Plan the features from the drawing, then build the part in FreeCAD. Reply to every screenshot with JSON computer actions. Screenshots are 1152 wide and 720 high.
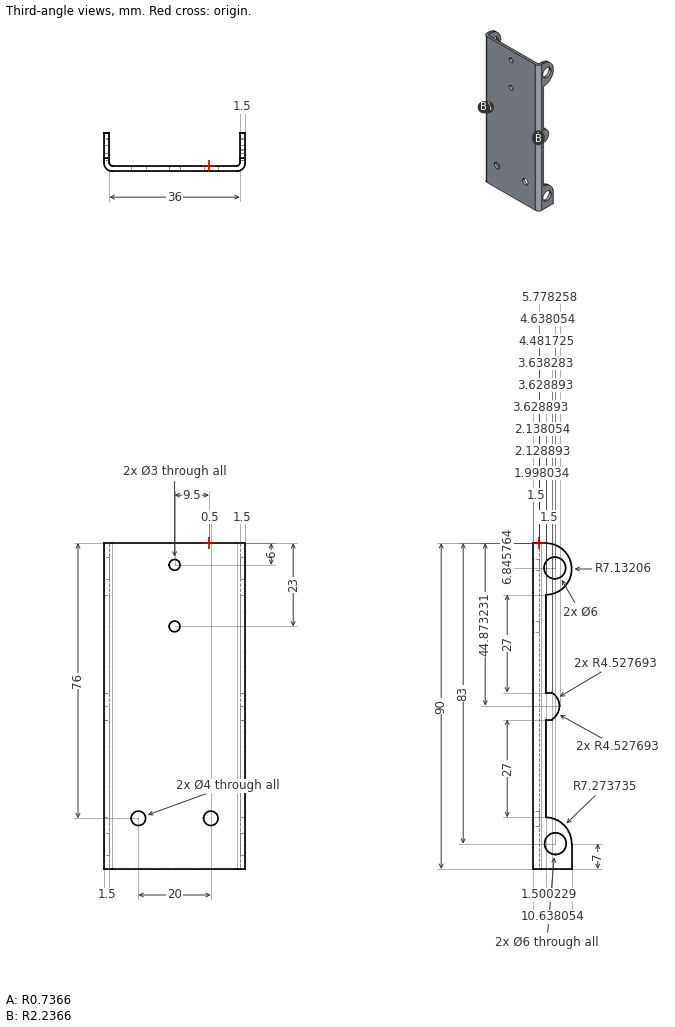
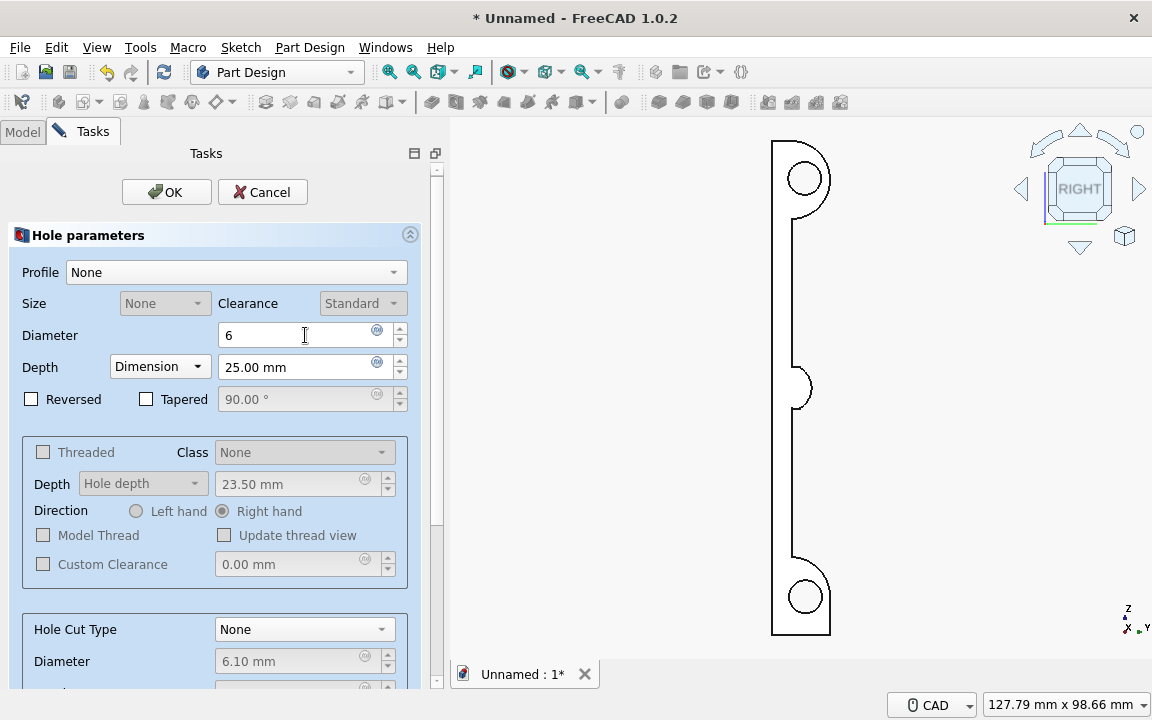
{"action": "left_click", "coordinate": [161, 366]}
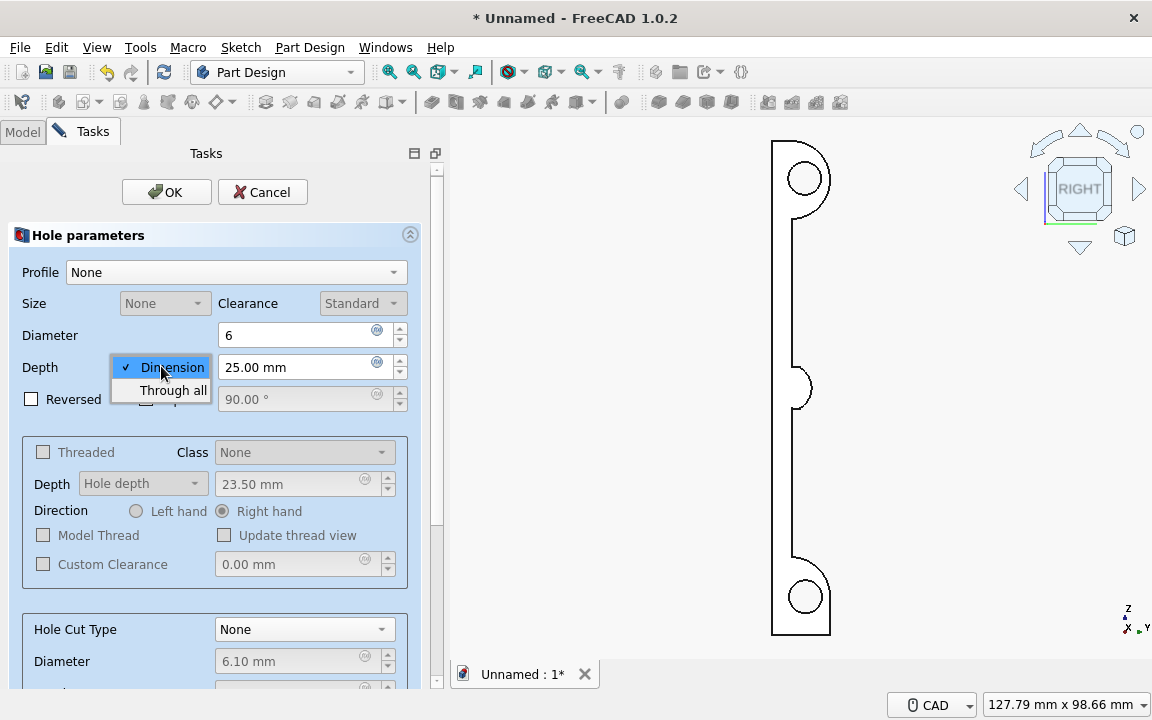
{"action": "left_click", "coordinate": [160, 390]}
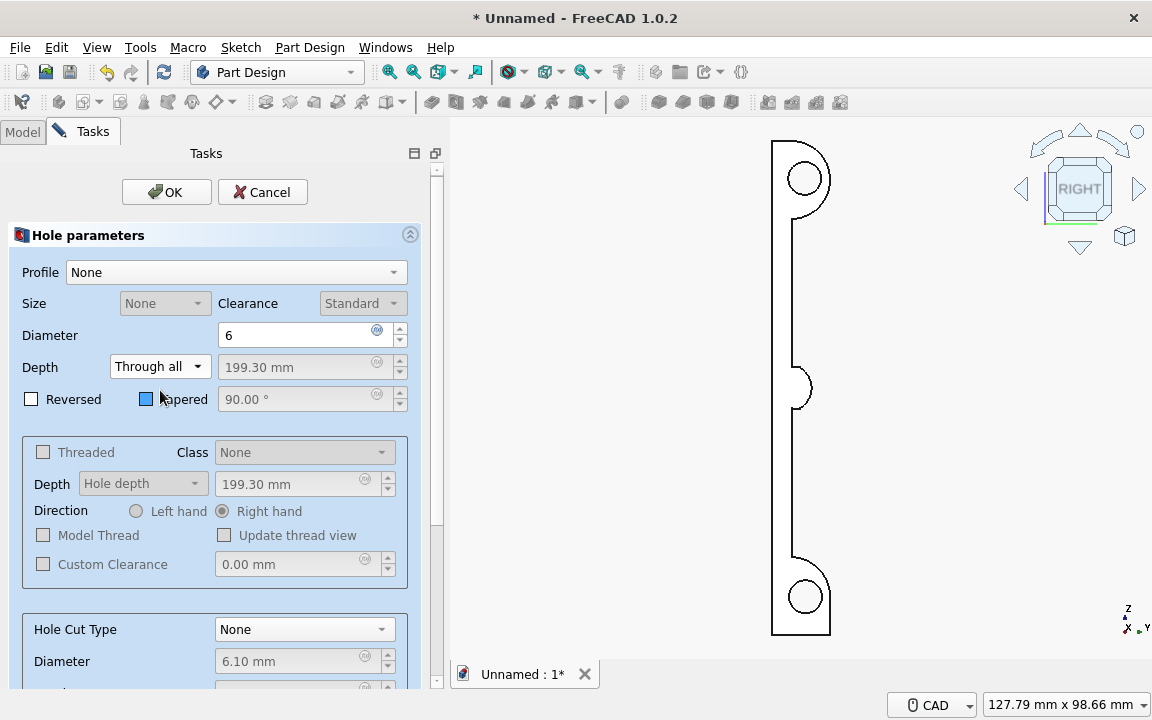
{"action": "left_click", "coordinate": [167, 192]}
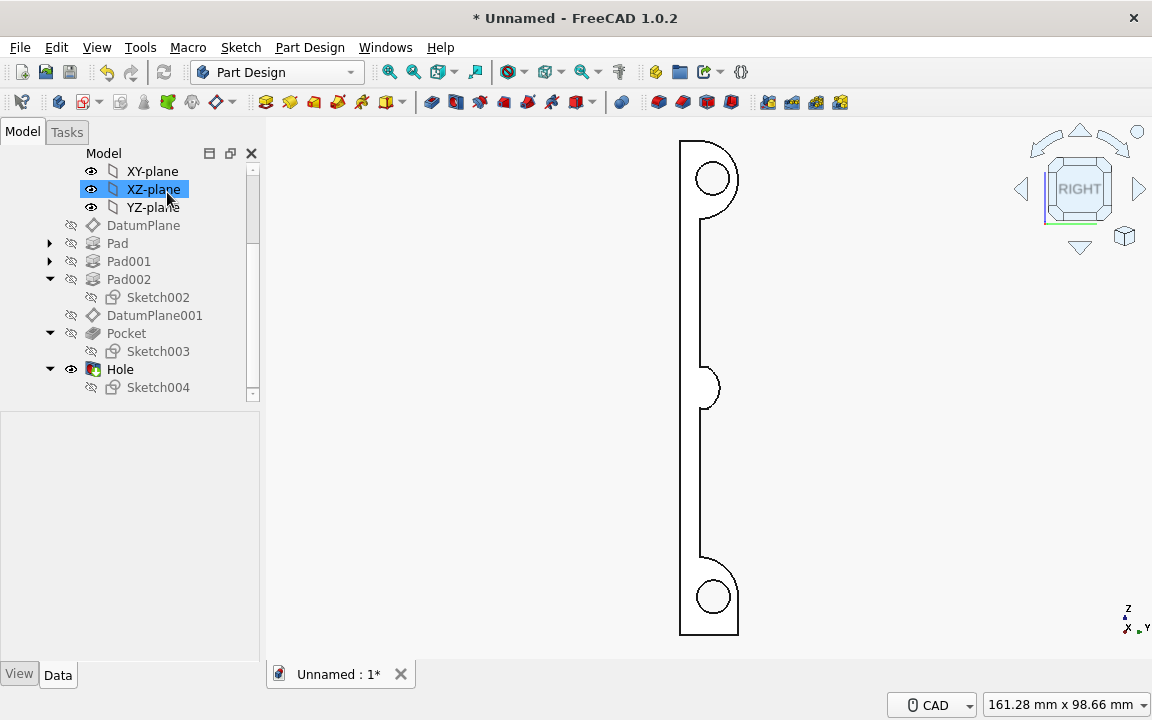
{"action": "left_click", "coordinate": [84, 102]}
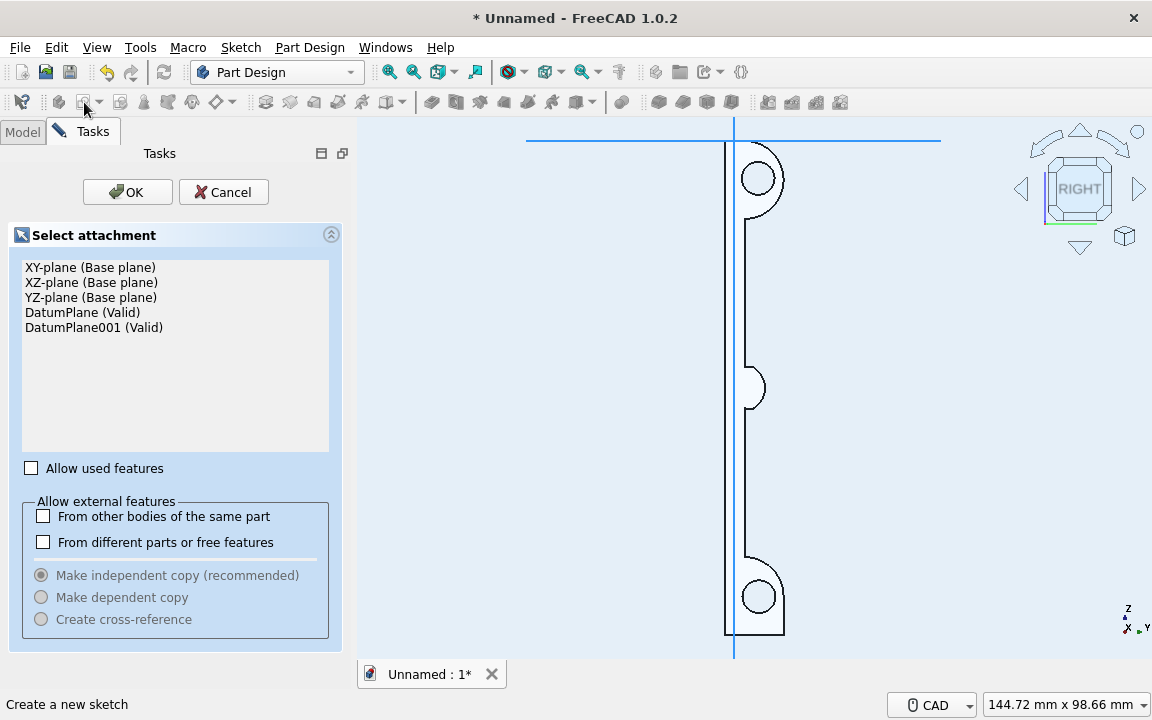
{"action": "left_click", "coordinate": [82, 282]}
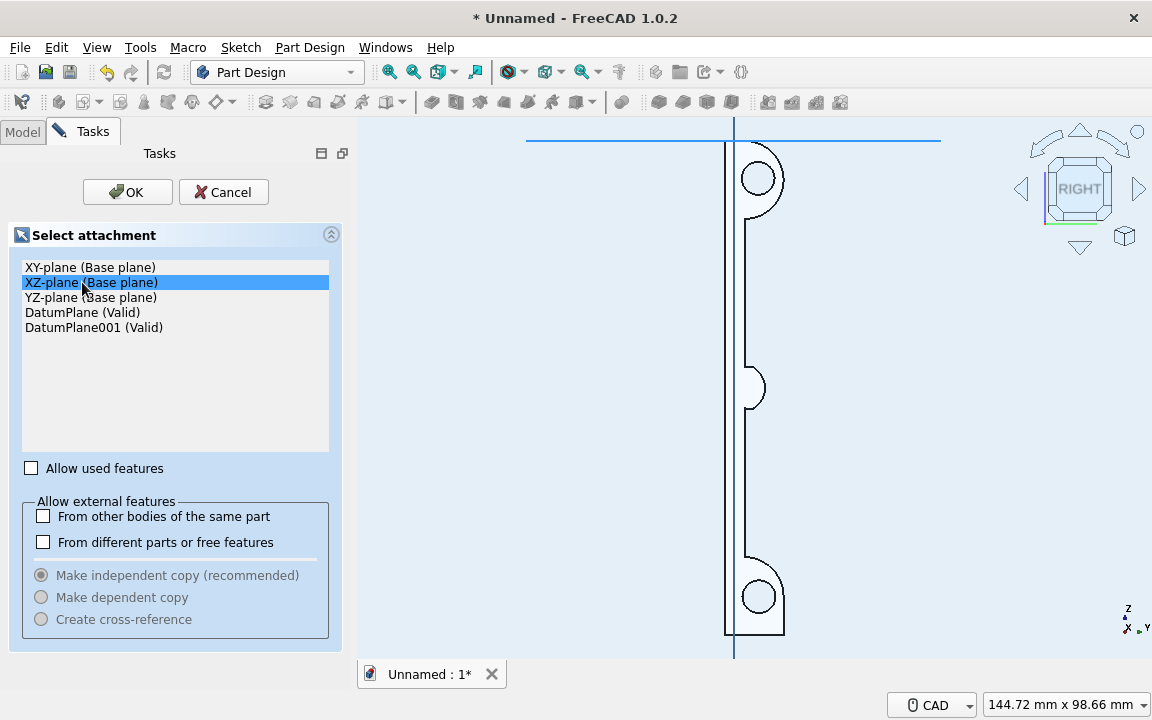
{"action": "left_click", "coordinate": [128, 192]}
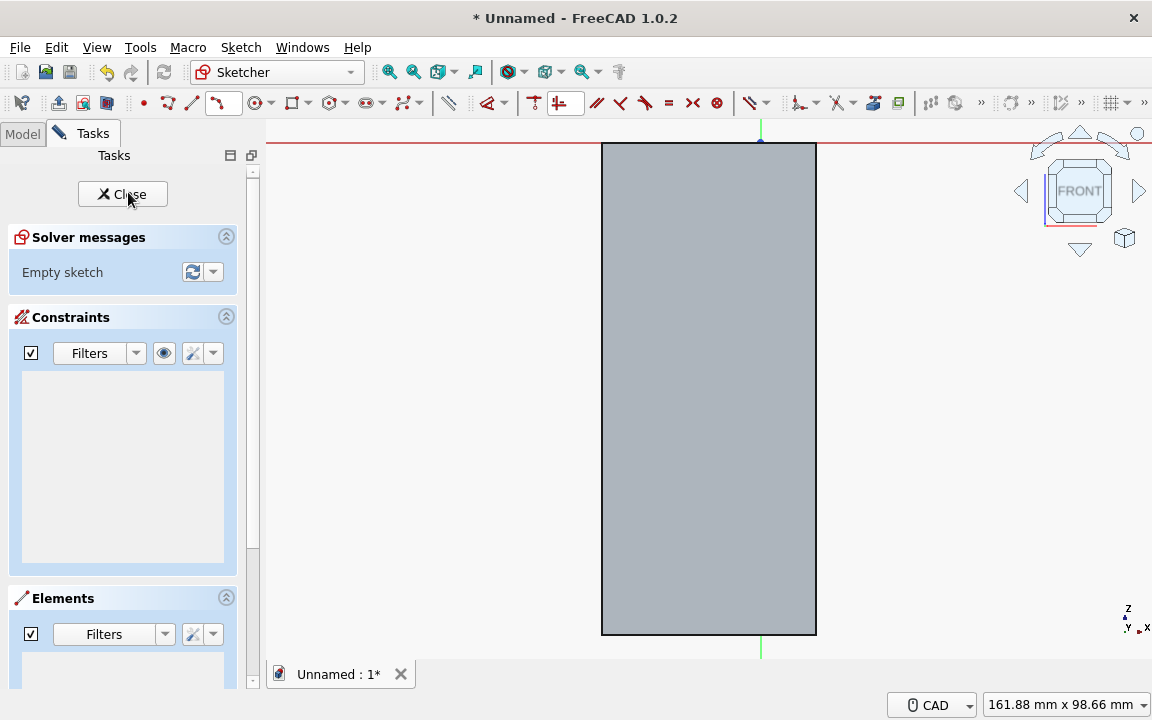
{"action": "key", "text": "q s"}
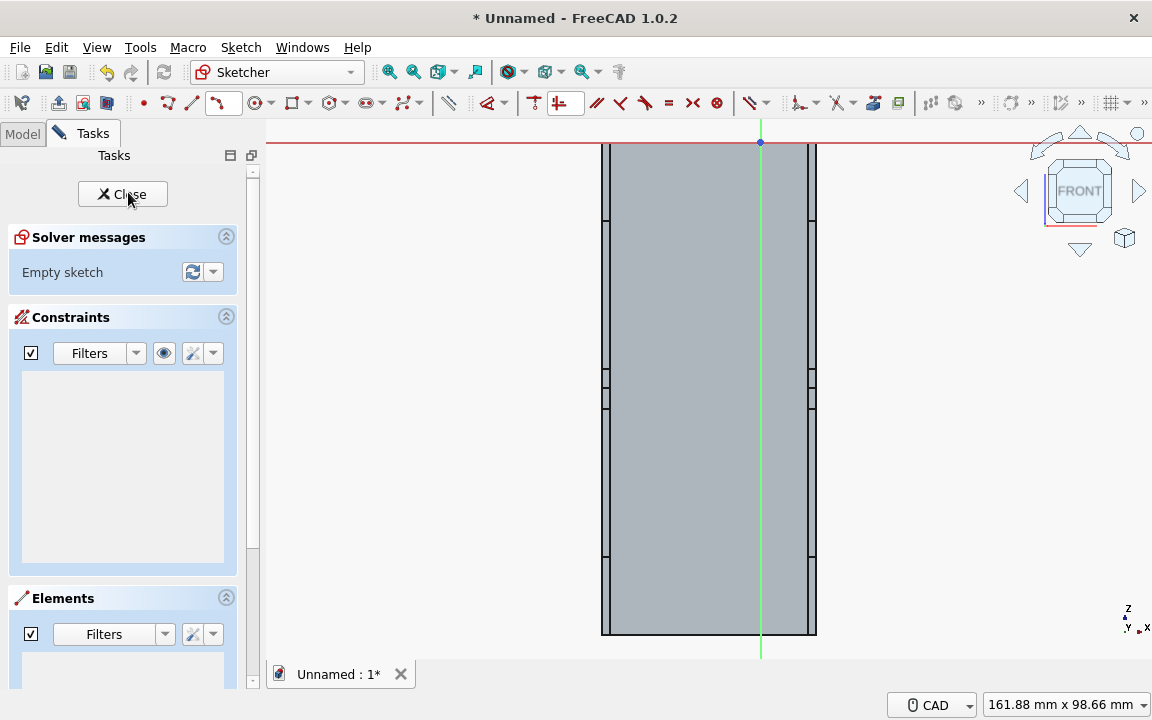
{"action": "scroll", "coordinate": [731, 614], "scroll_direction": "up", "scroll_amount": 7}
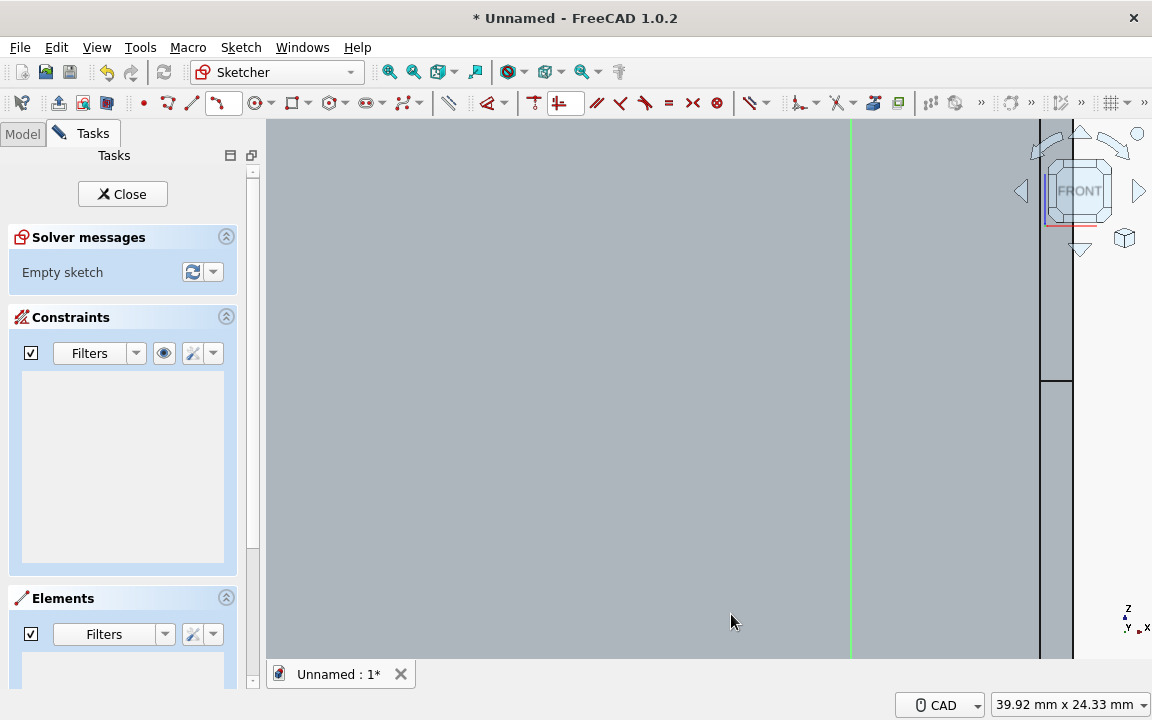
{"action": "left_click", "coordinate": [256, 104]}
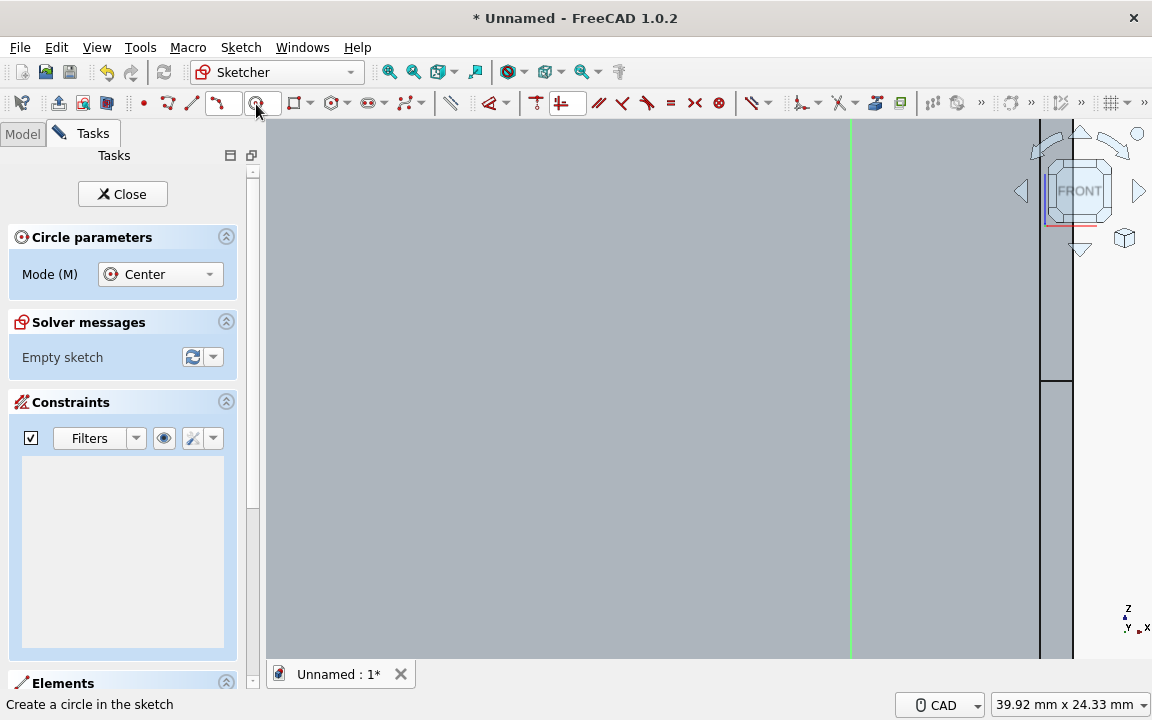
{"action": "left_click", "coordinate": [418, 387]}
{"action": "left_click", "coordinate": [450, 355]}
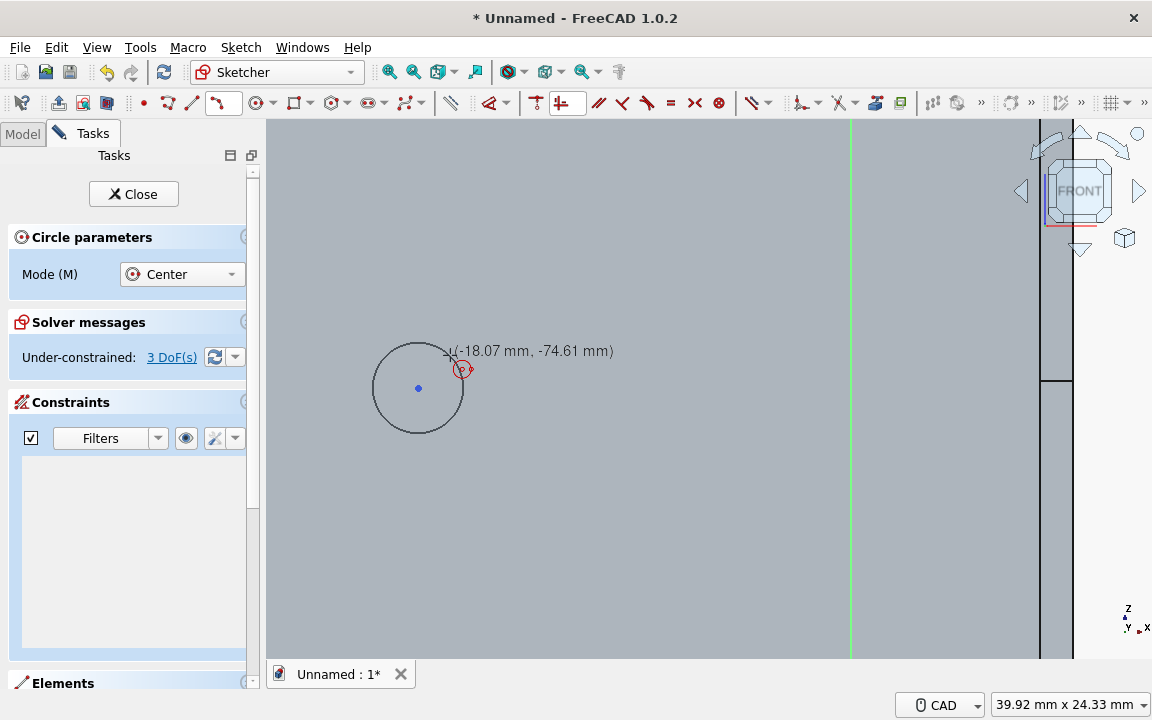
{"action": "scroll", "coordinate": [862, 387], "scroll_direction": "up", "scroll_amount": 2}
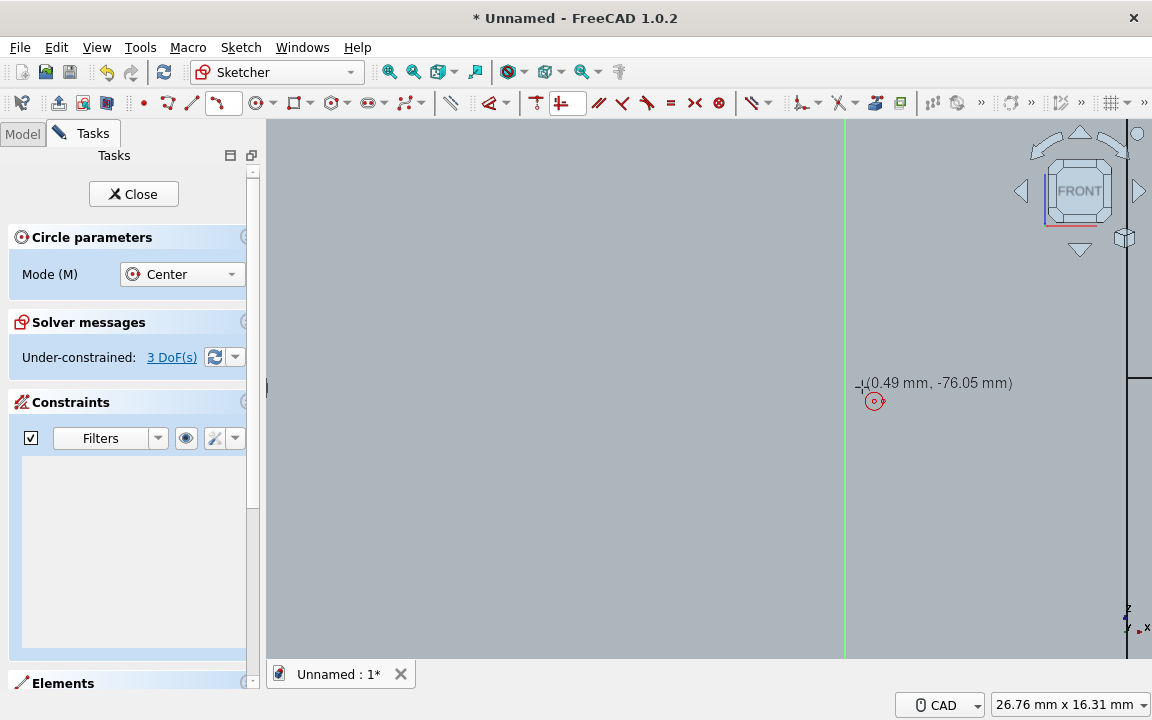
{"action": "left_click", "coordinate": [862, 386]}
{"action": "left_click", "coordinate": [909, 340]}
{"action": "key", "text": "Escape"}